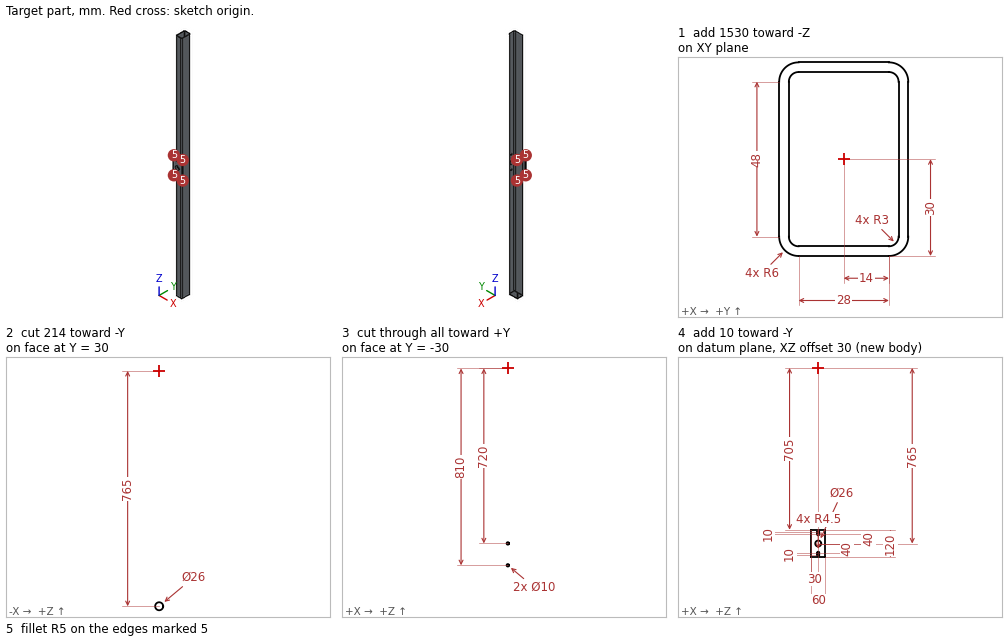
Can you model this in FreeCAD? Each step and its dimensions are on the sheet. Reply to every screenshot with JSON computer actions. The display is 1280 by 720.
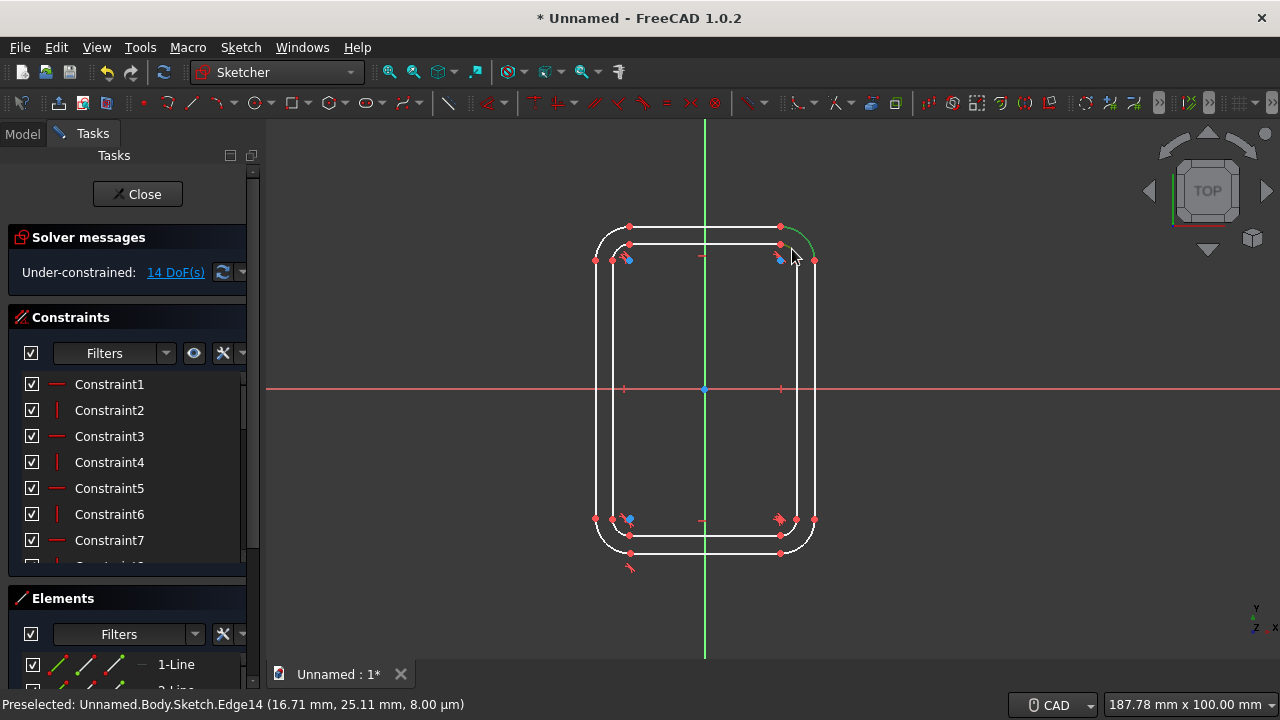
{"action": "left_click", "coordinate": [534, 104]}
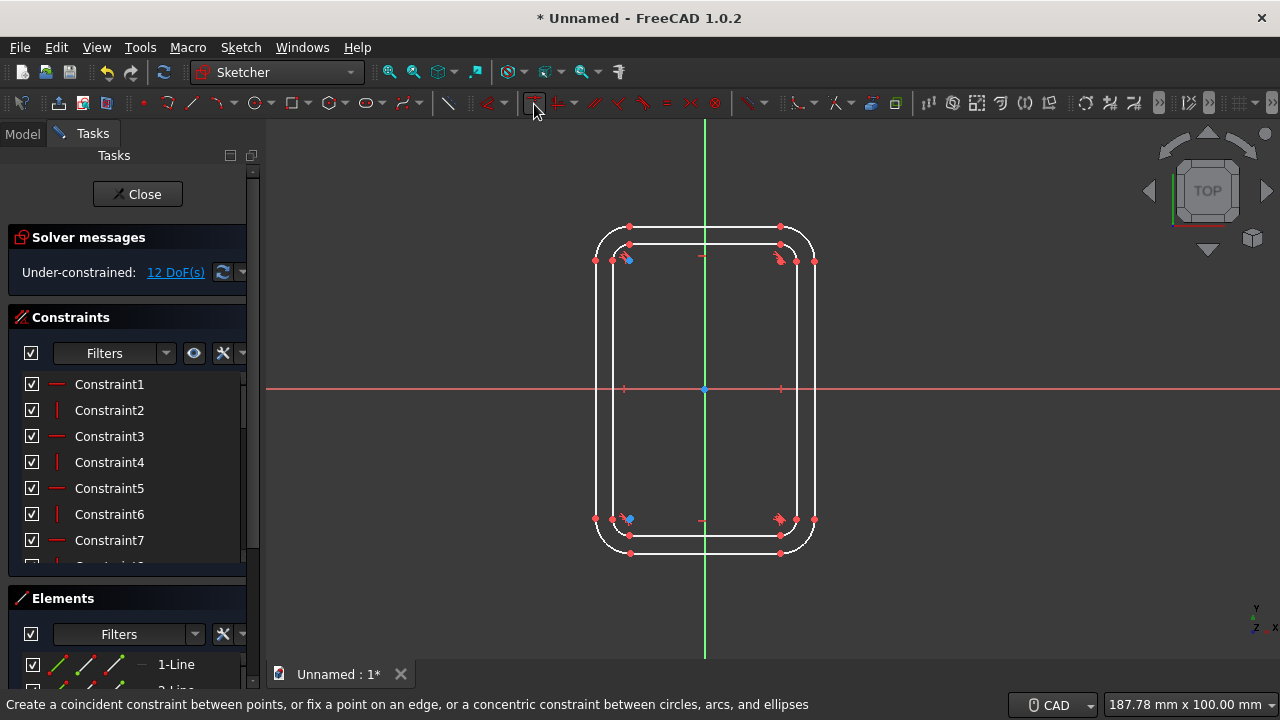
{"action": "left_click", "coordinate": [614, 230]}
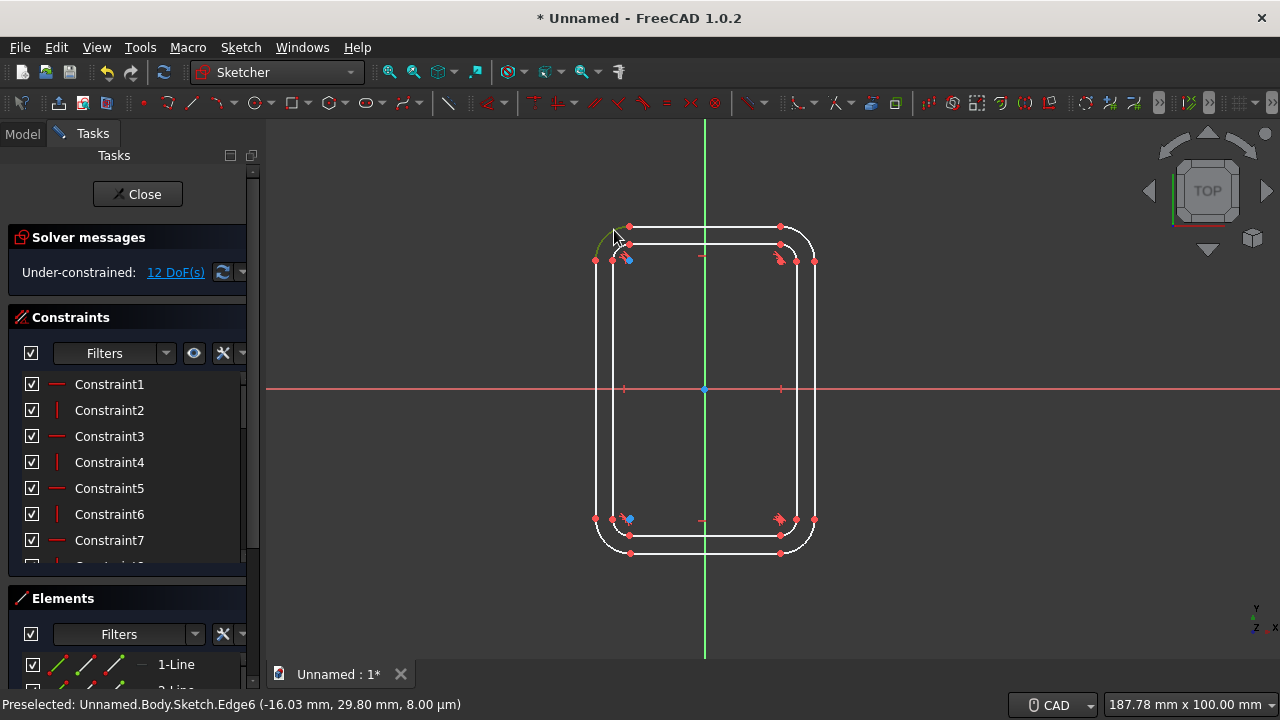
{"action": "left_click", "coordinate": [618, 249]}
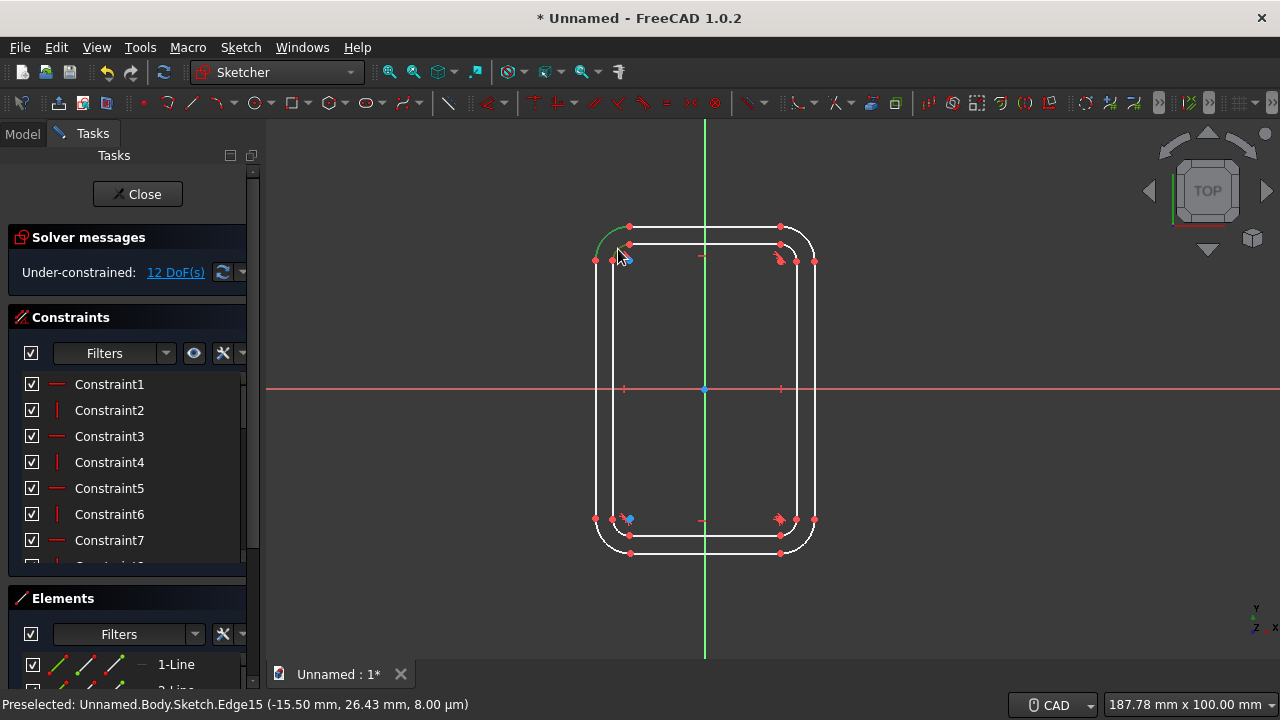
{"action": "left_click", "coordinate": [534, 104]}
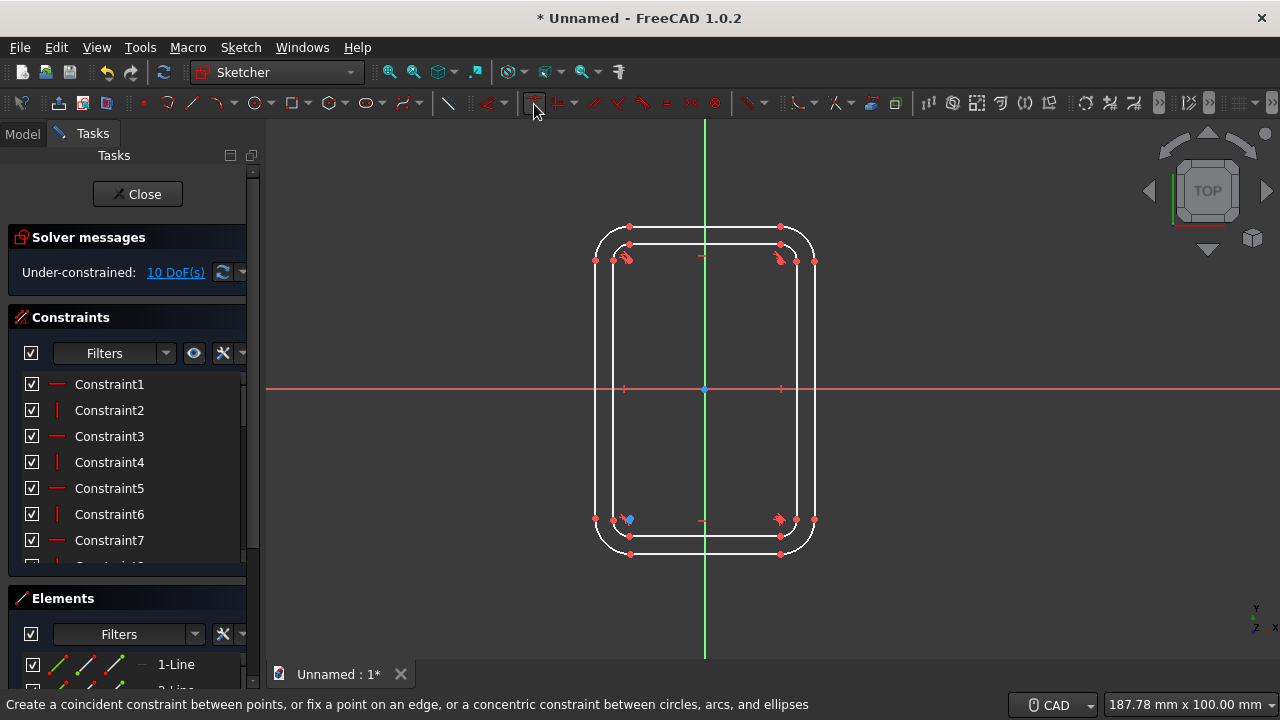
{"action": "left_click", "coordinate": [599, 535]}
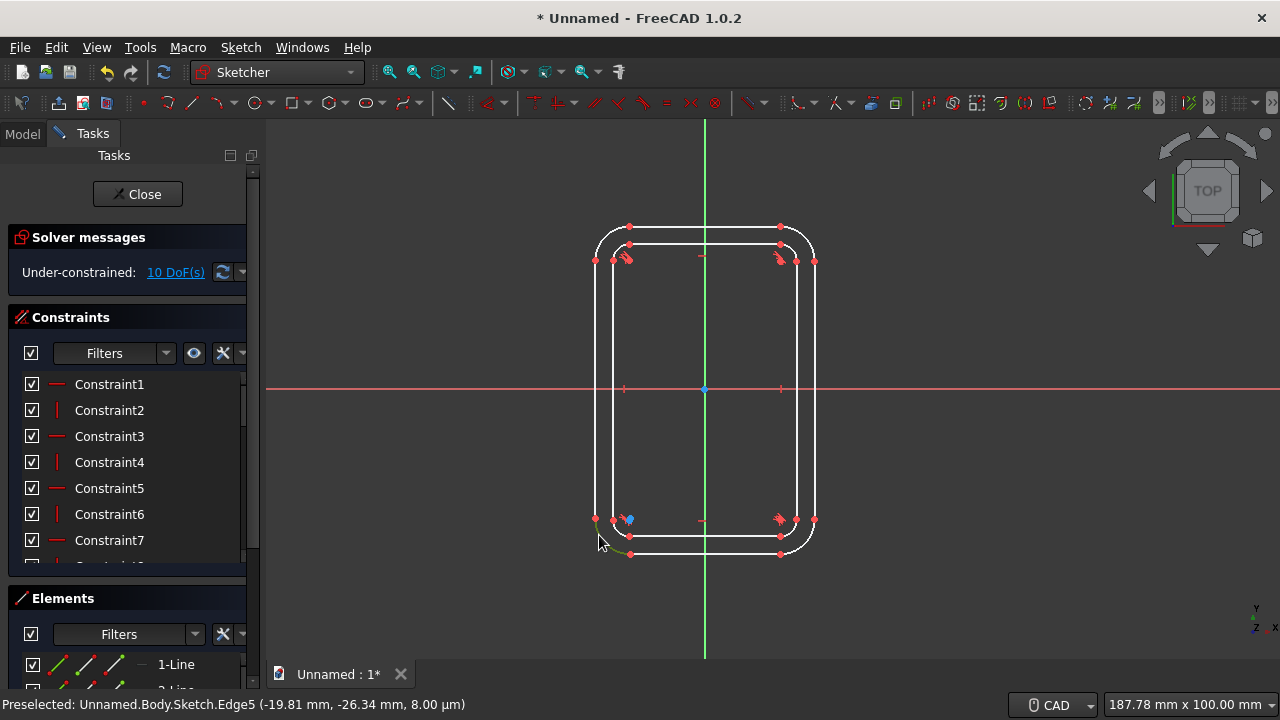
{"action": "left_click", "coordinate": [614, 230]}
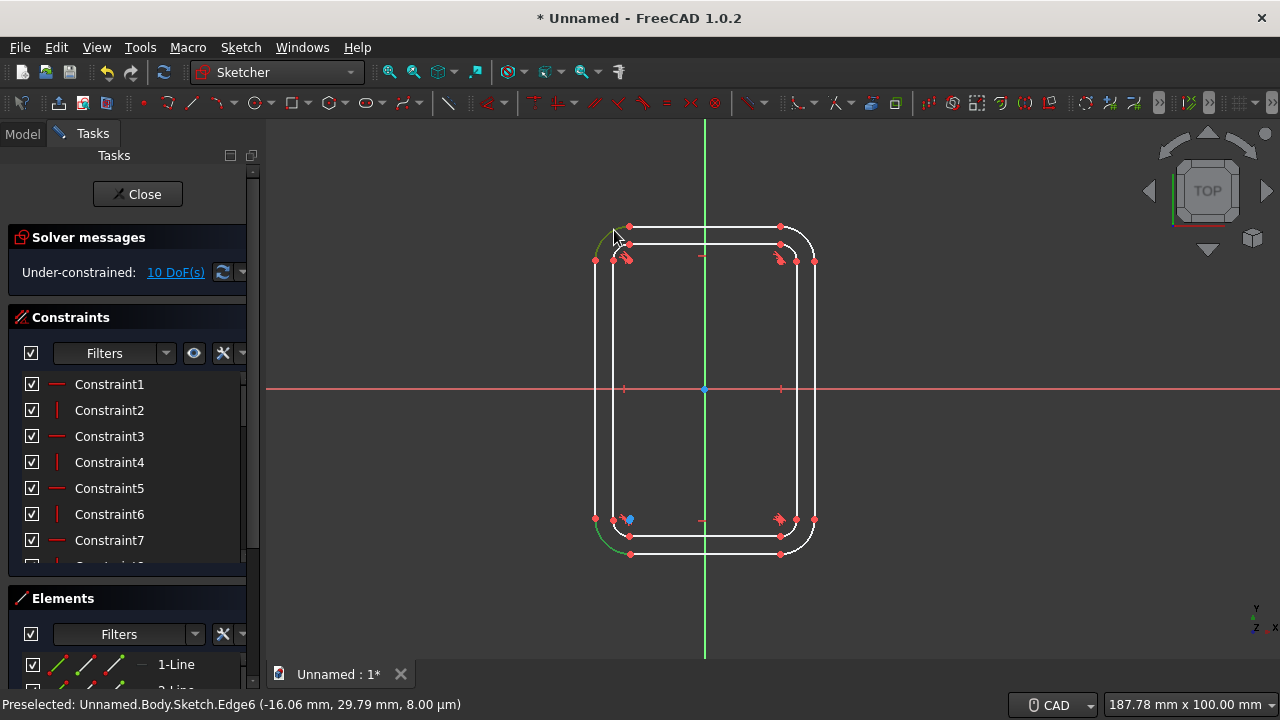
{"action": "left_click", "coordinate": [811, 245]}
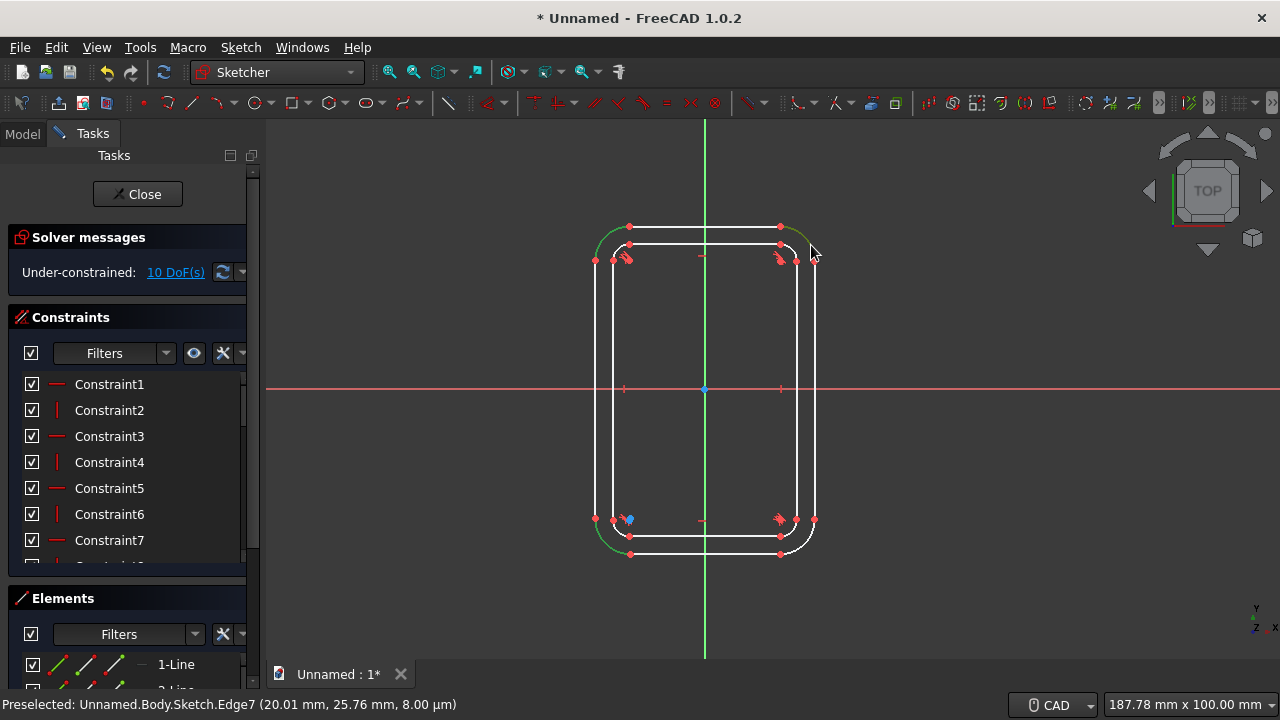
{"action": "left_click", "coordinate": [796, 550]}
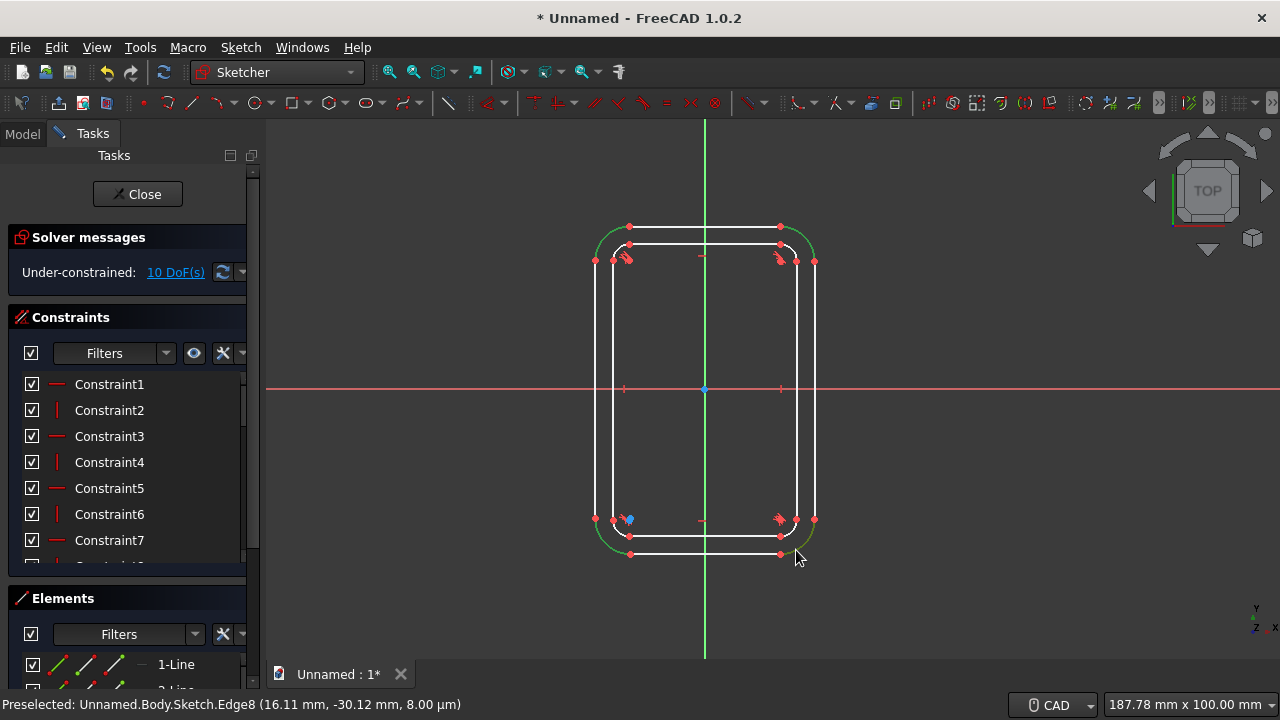
{"action": "left_click", "coordinate": [668, 104]}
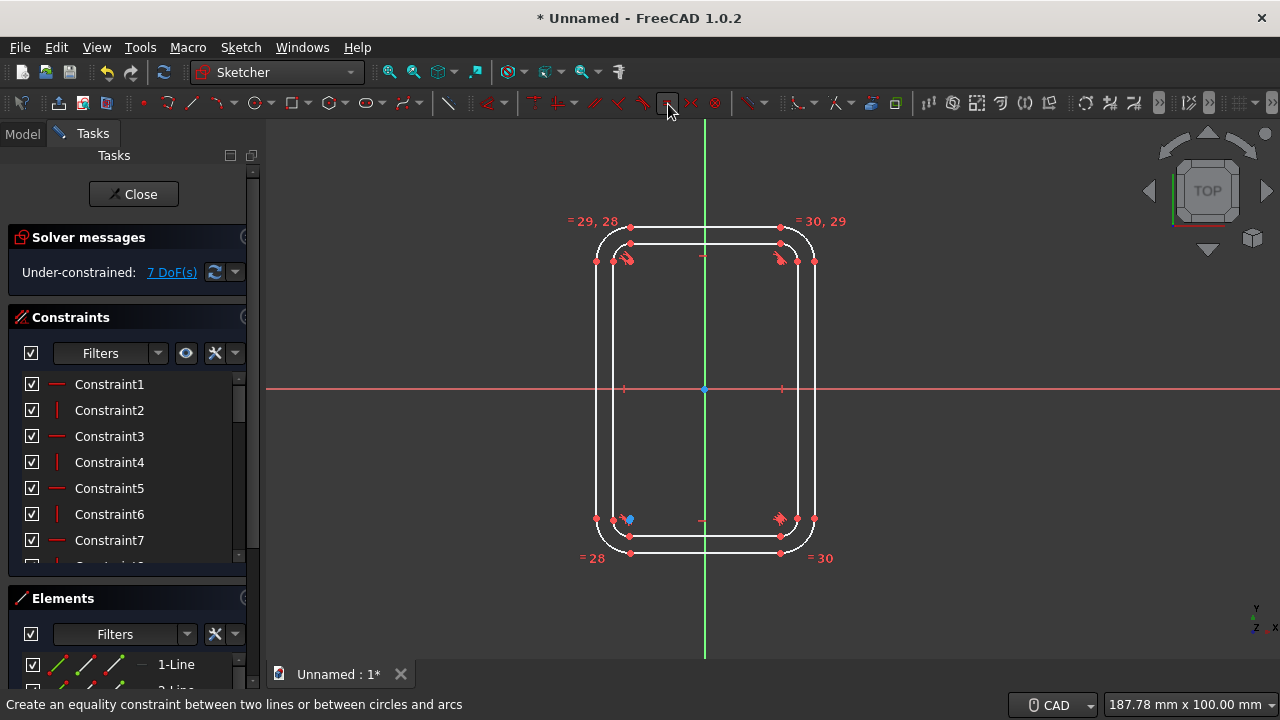
{"action": "left_click", "coordinate": [793, 531]}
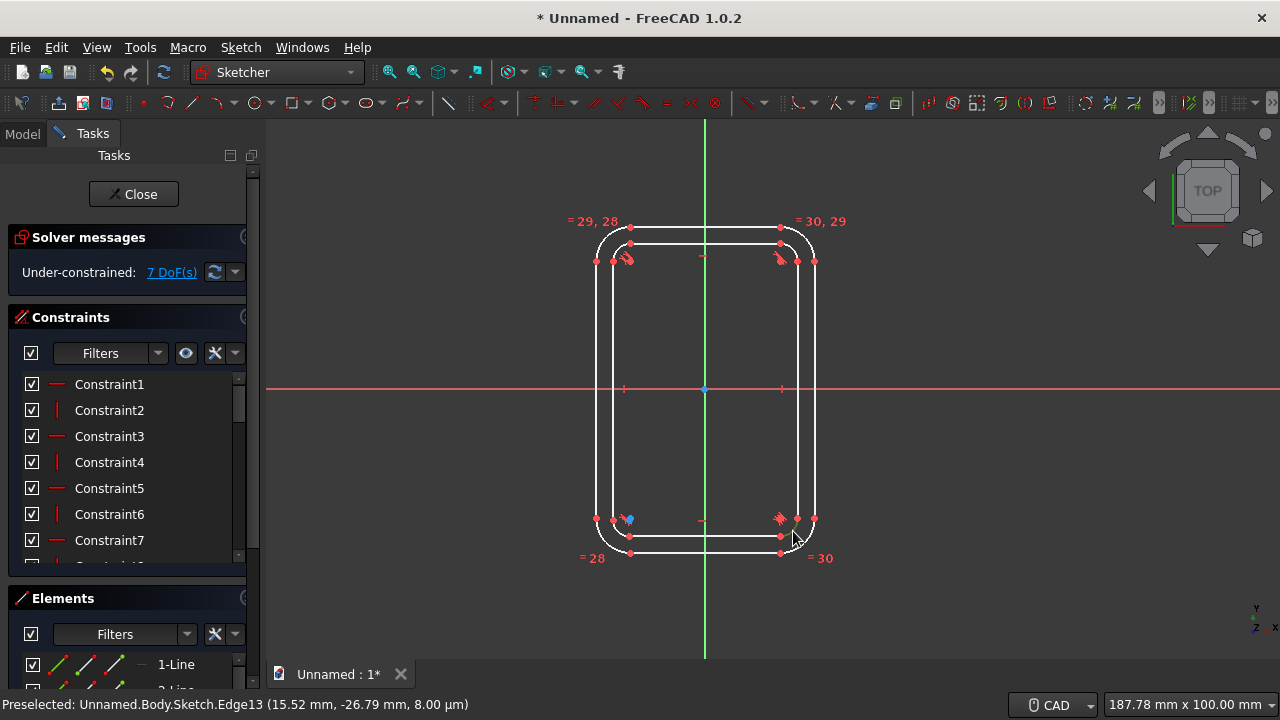
{"action": "left_click", "coordinate": [618, 532]}